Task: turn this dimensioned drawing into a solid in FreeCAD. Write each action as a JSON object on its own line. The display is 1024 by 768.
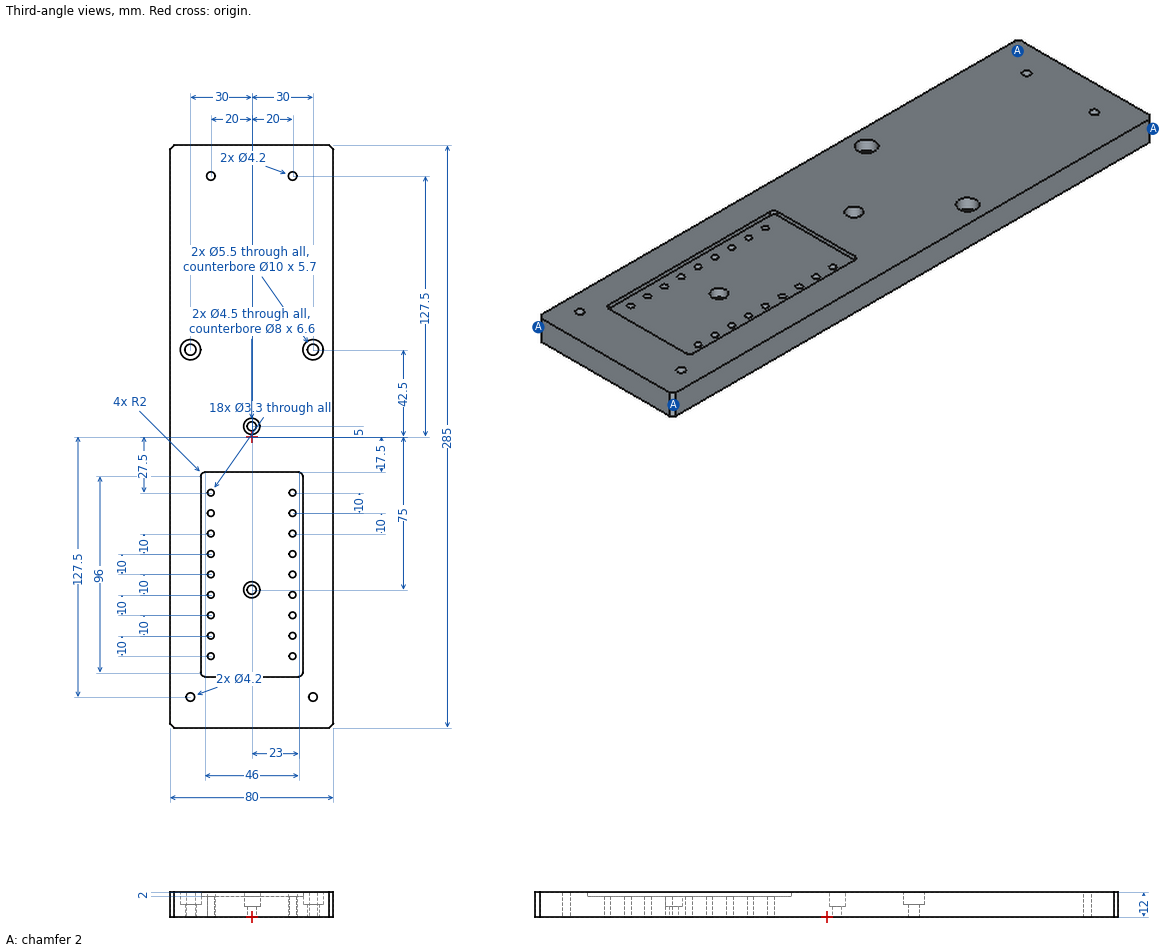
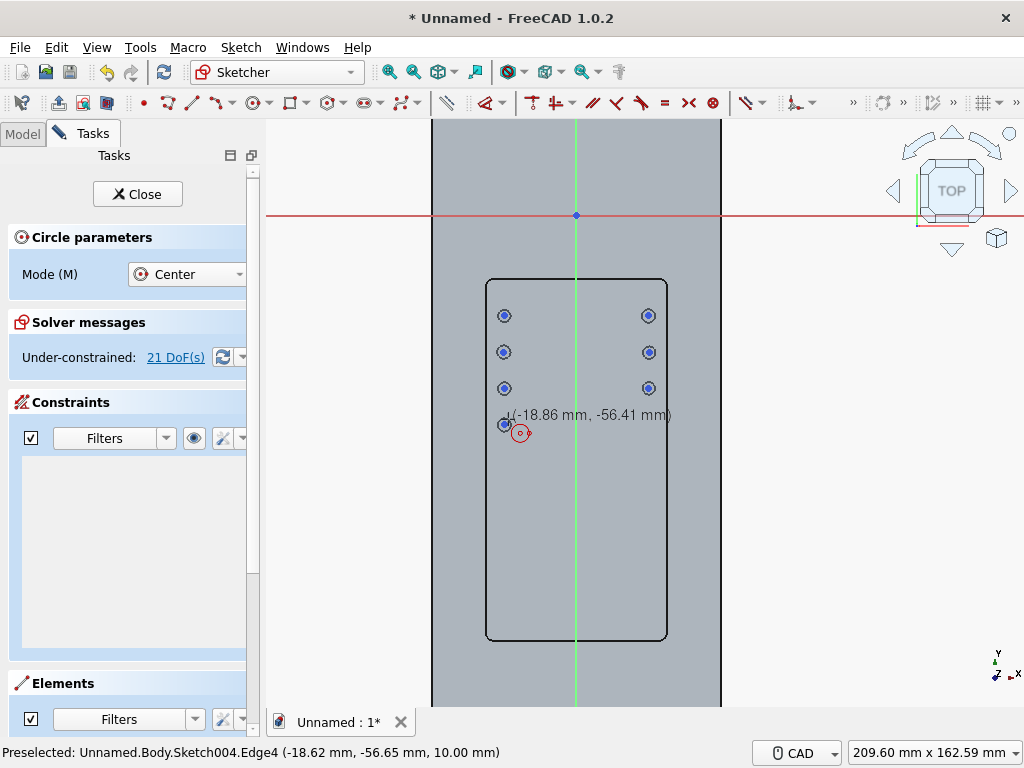
{"action": "scroll", "coordinate": [649, 424], "scroll_direction": "up", "scroll_amount": 7}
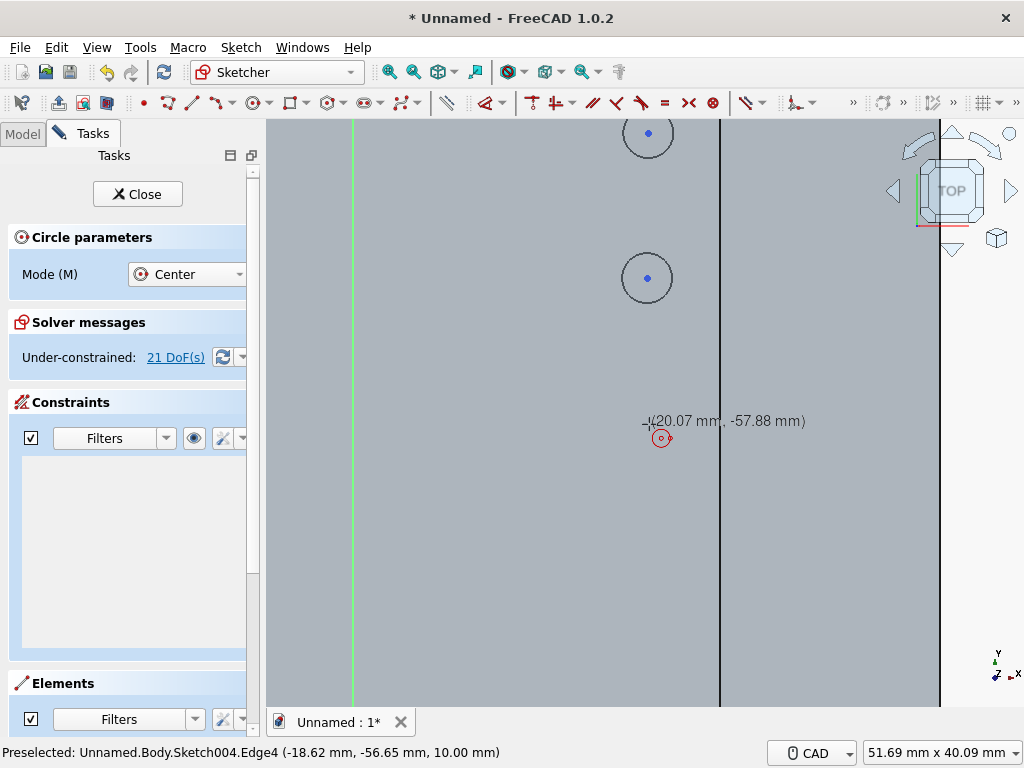
{"action": "scroll", "coordinate": [650, 424], "scroll_direction": "down", "scroll_amount": 7}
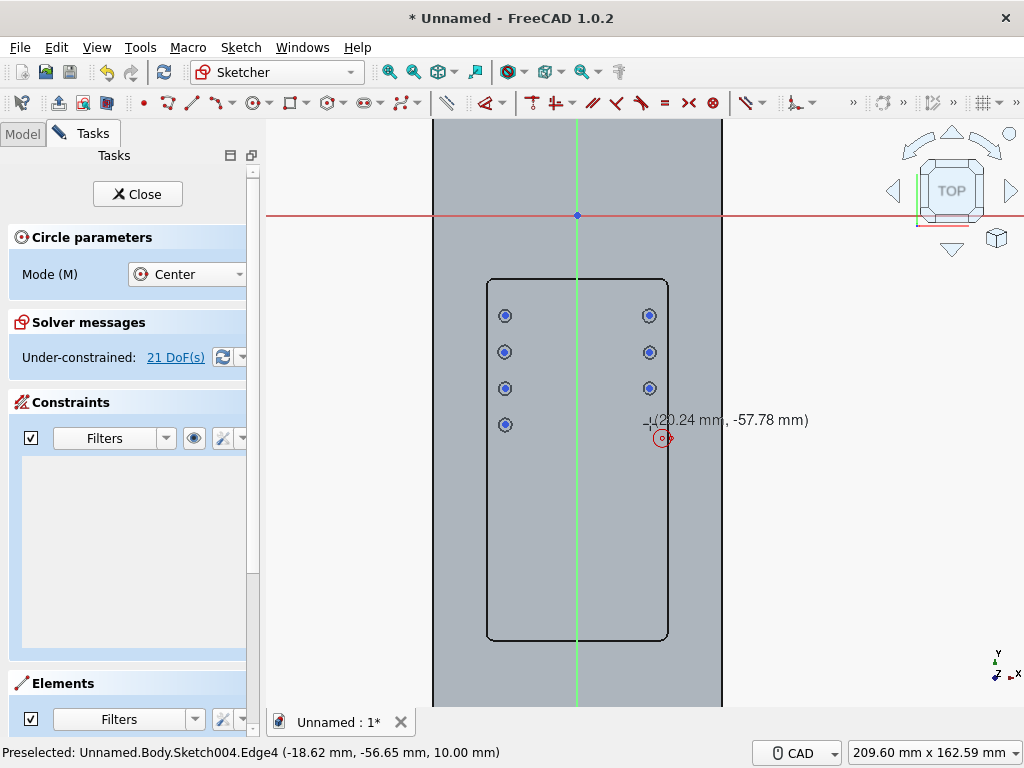
{"action": "left_click", "coordinate": [650, 424]}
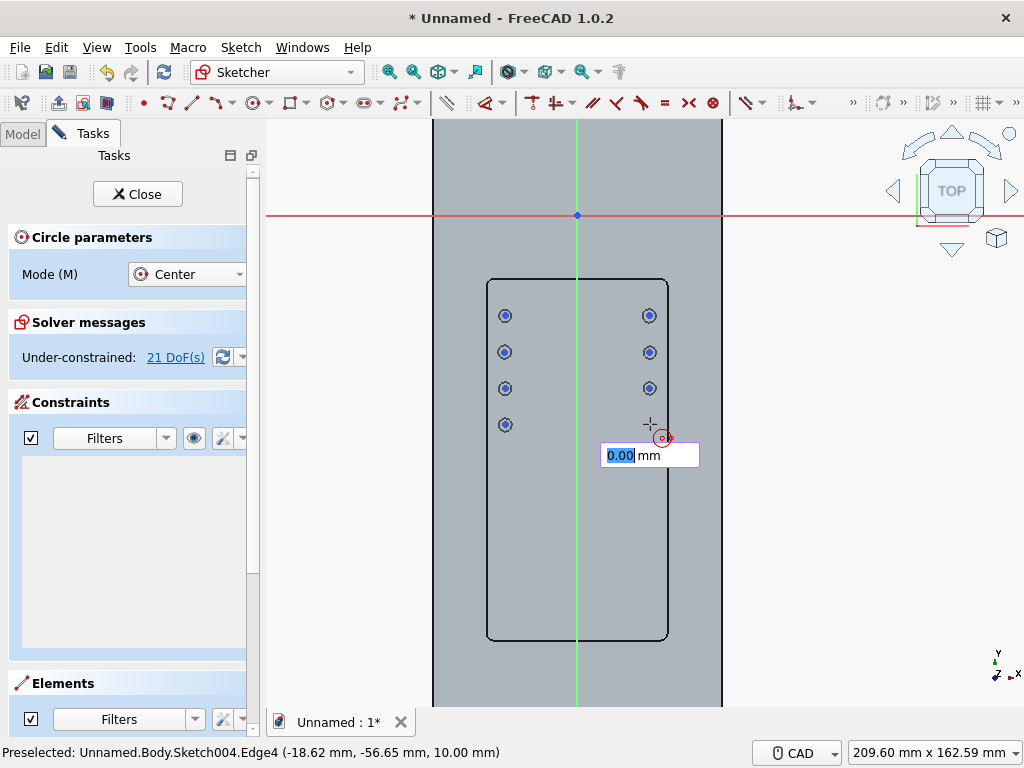
{"action": "scroll", "coordinate": [654, 419], "scroll_direction": "up", "scroll_amount": 5}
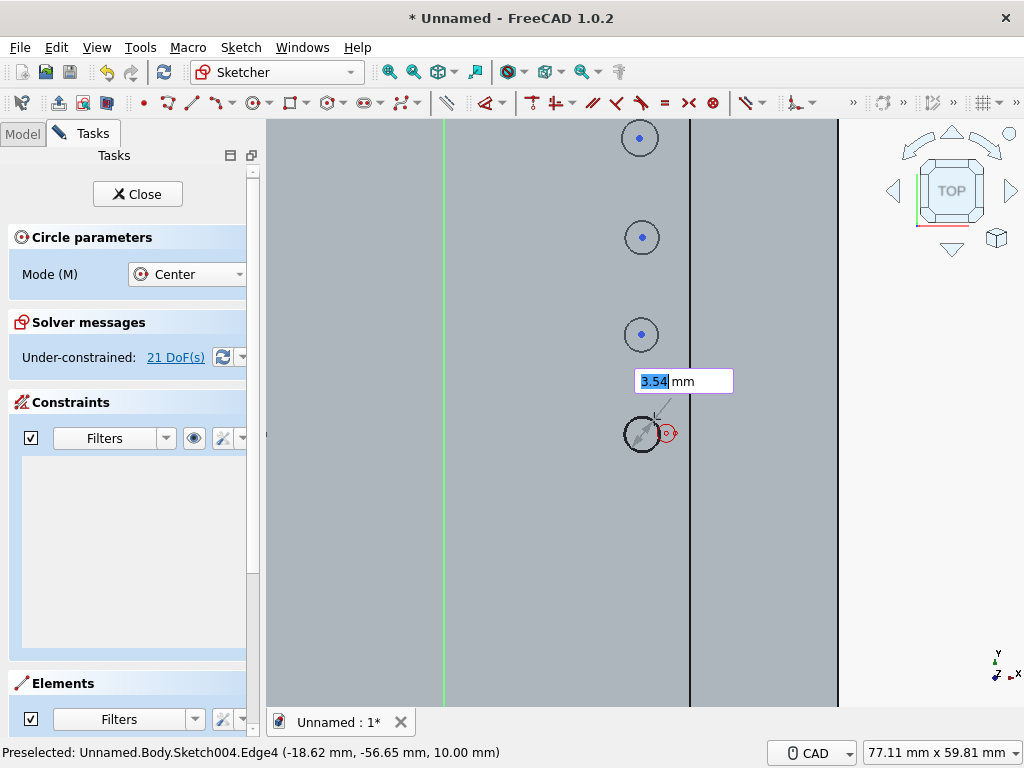
{"action": "left_click", "coordinate": [652, 419]}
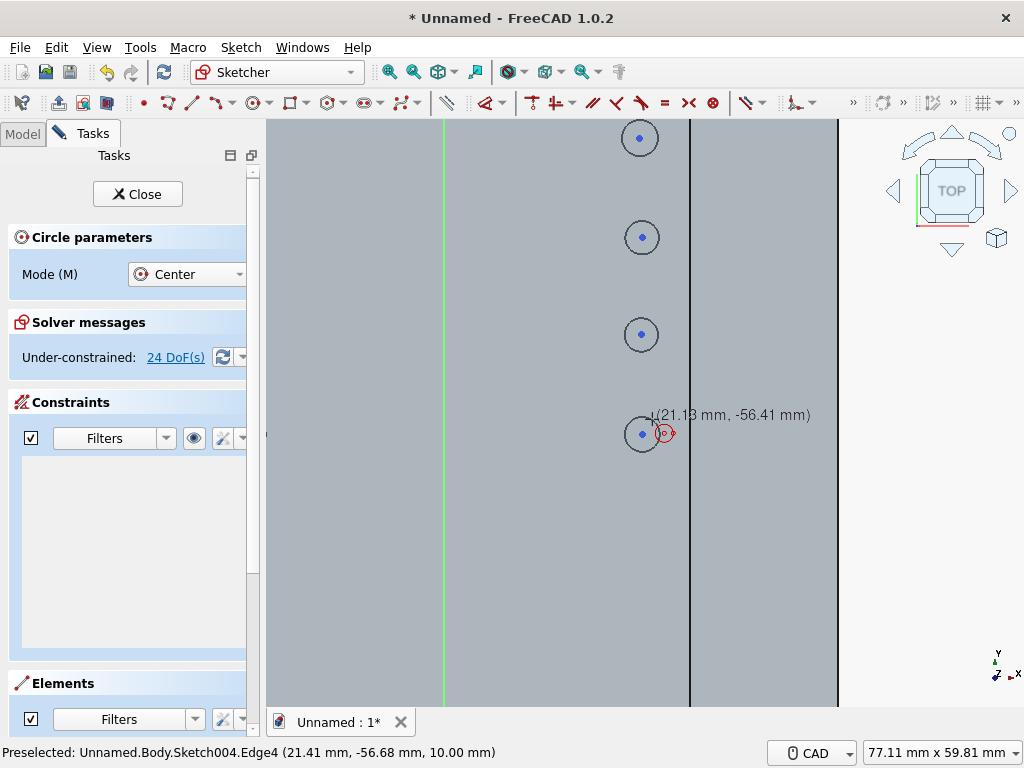
{"action": "scroll", "coordinate": [653, 419], "scroll_direction": "down", "scroll_amount": 5}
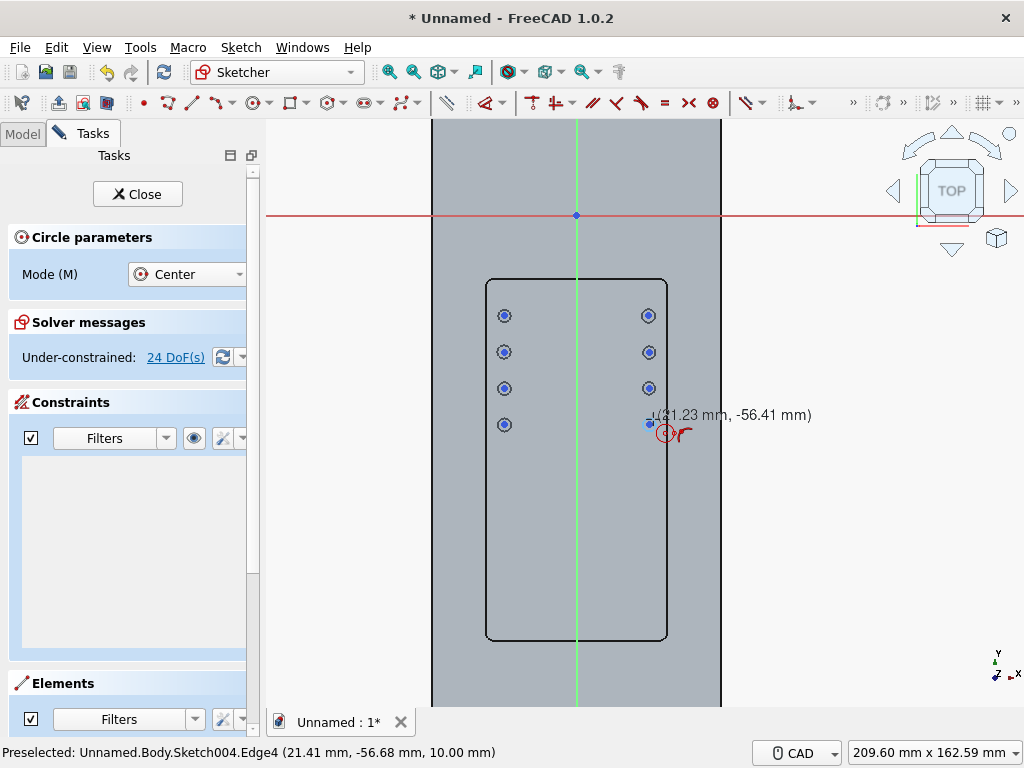
{"action": "scroll", "coordinate": [504, 460], "scroll_direction": "up", "scroll_amount": 7}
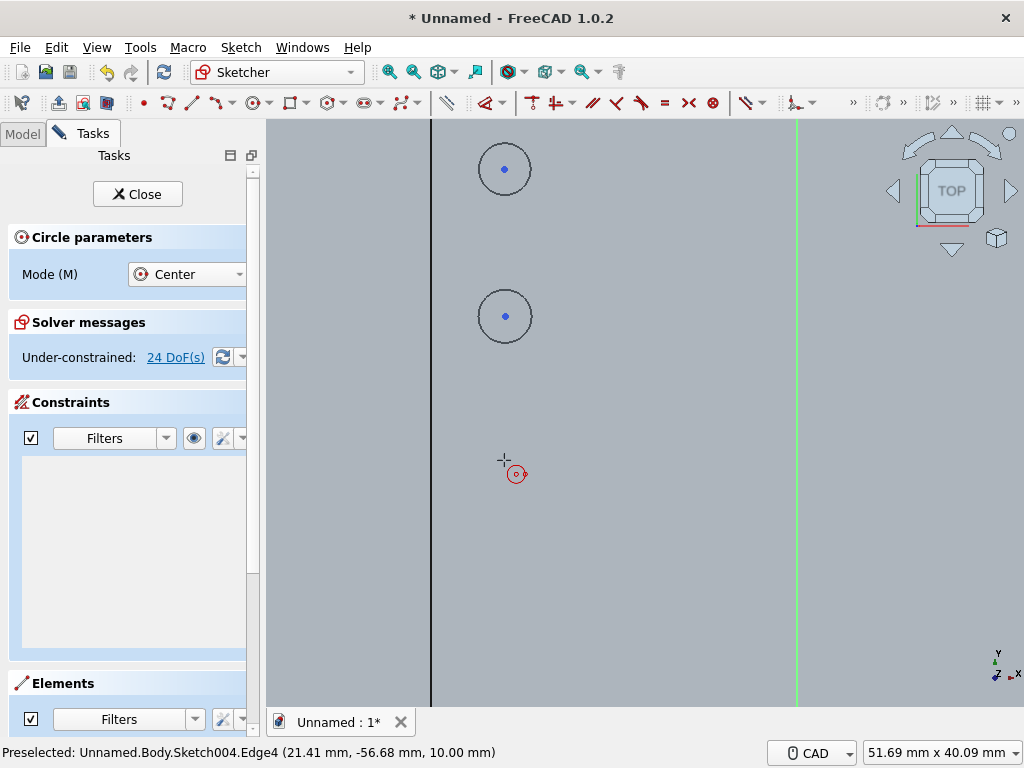
{"action": "scroll", "coordinate": [504, 461], "scroll_direction": "down", "scroll_amount": 7}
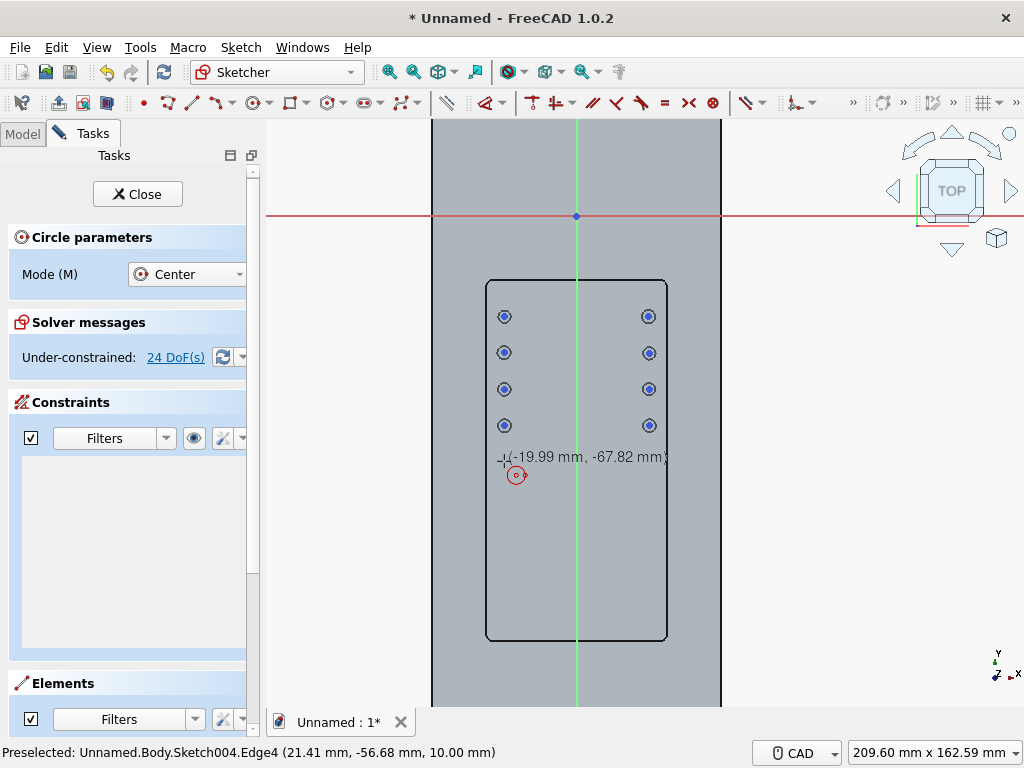
{"action": "left_click", "coordinate": [504, 461]}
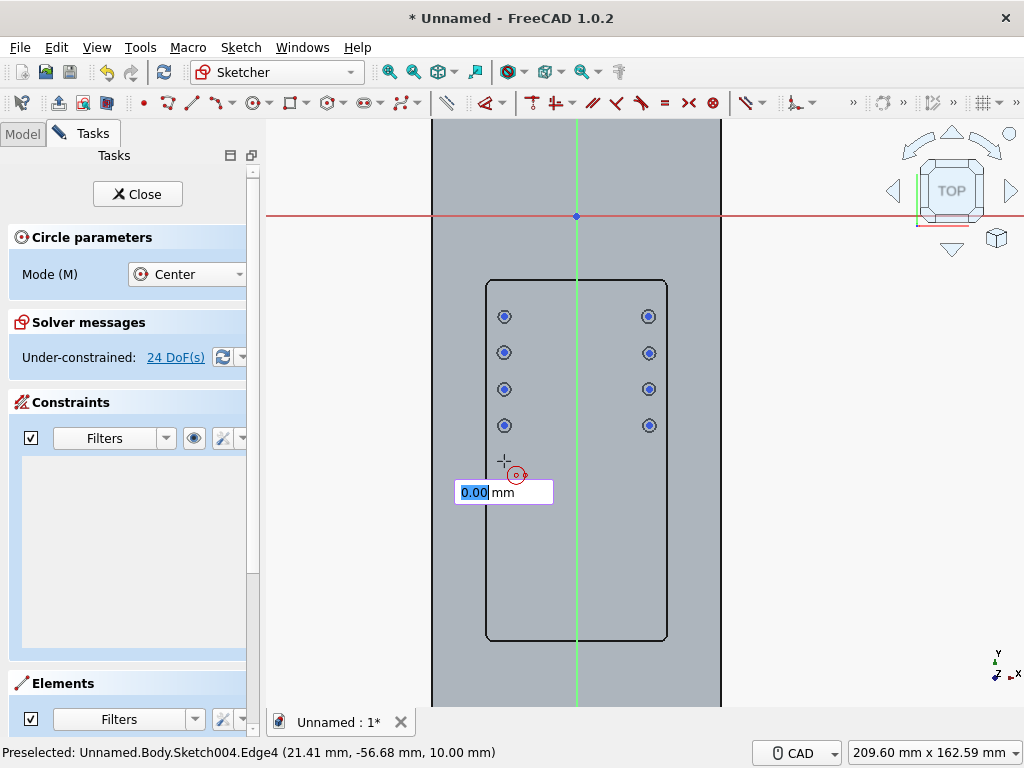
{"action": "scroll", "coordinate": [508, 456], "scroll_direction": "up", "scroll_amount": 5}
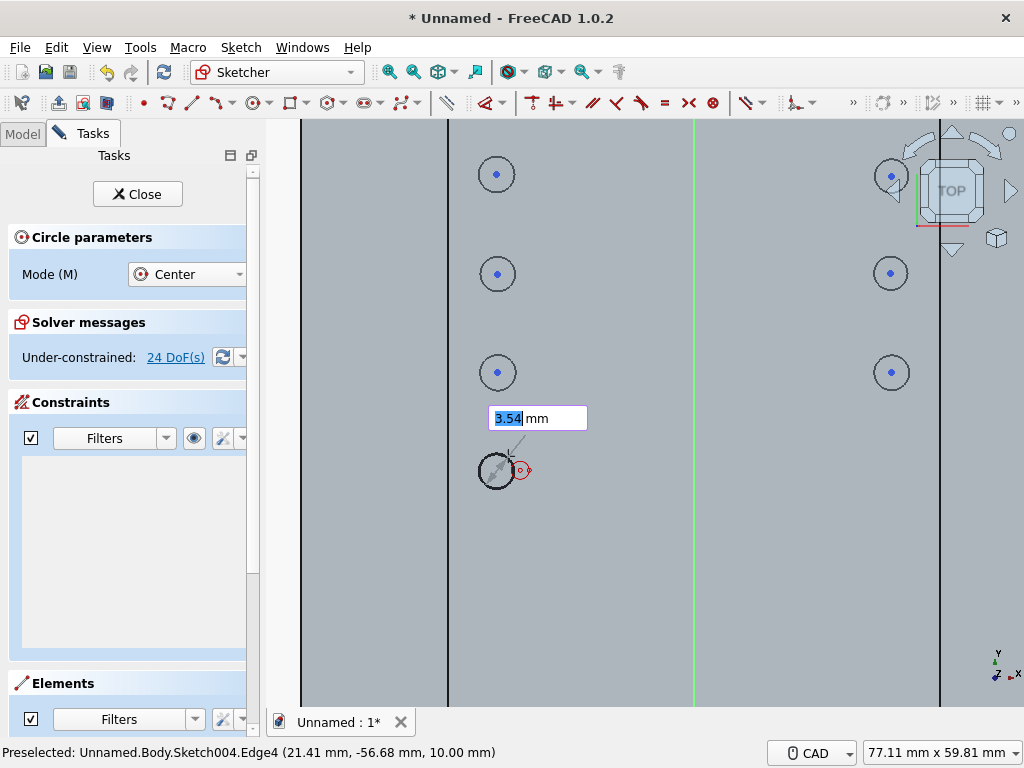
{"action": "left_click", "coordinate": [509, 456]}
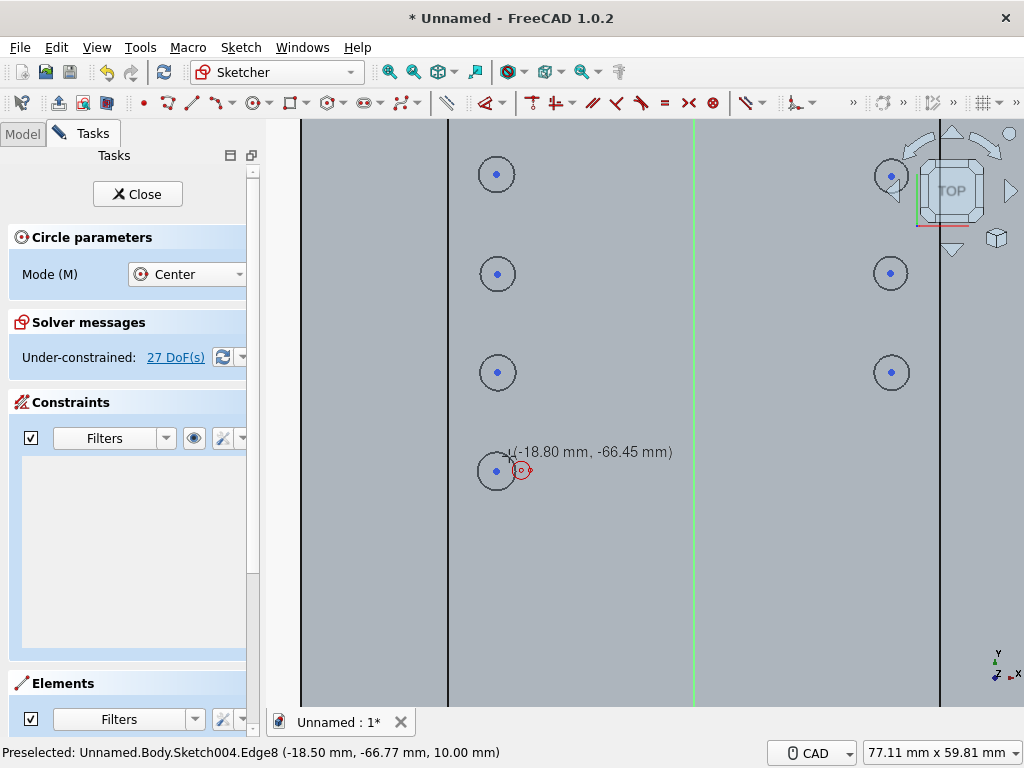
{"action": "scroll", "coordinate": [508, 455], "scroll_direction": "down", "scroll_amount": 5}